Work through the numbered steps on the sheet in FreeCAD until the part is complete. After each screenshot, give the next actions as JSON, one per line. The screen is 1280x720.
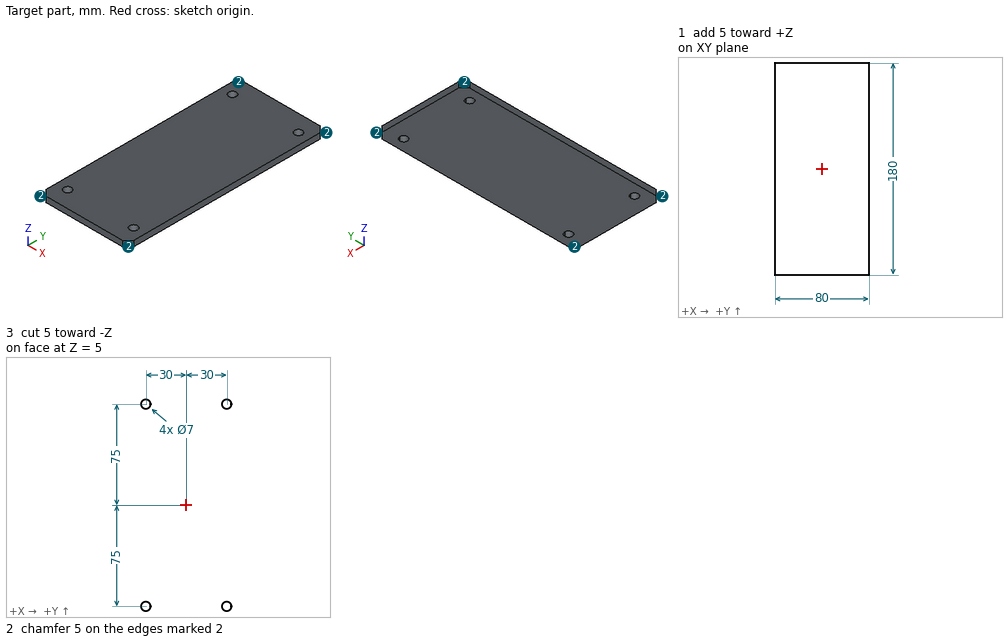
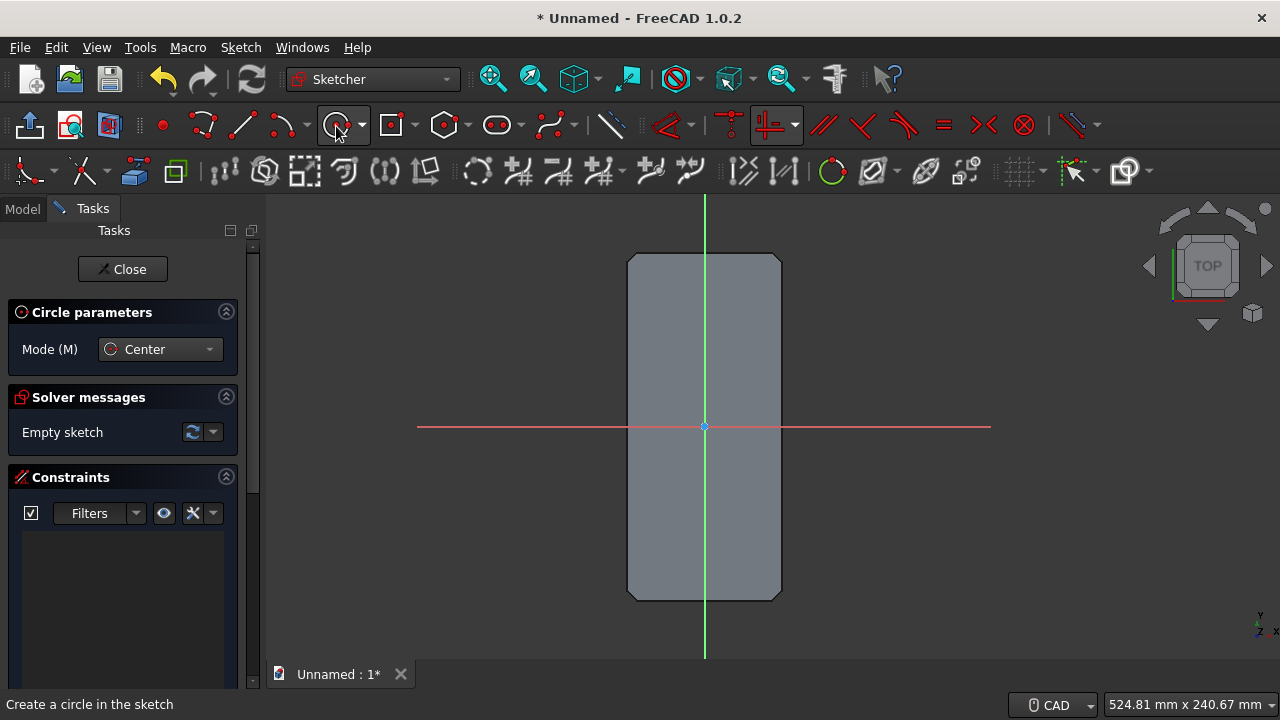
{"action": "scroll", "coordinate": [647, 282], "scroll_direction": "up", "scroll_amount": 7}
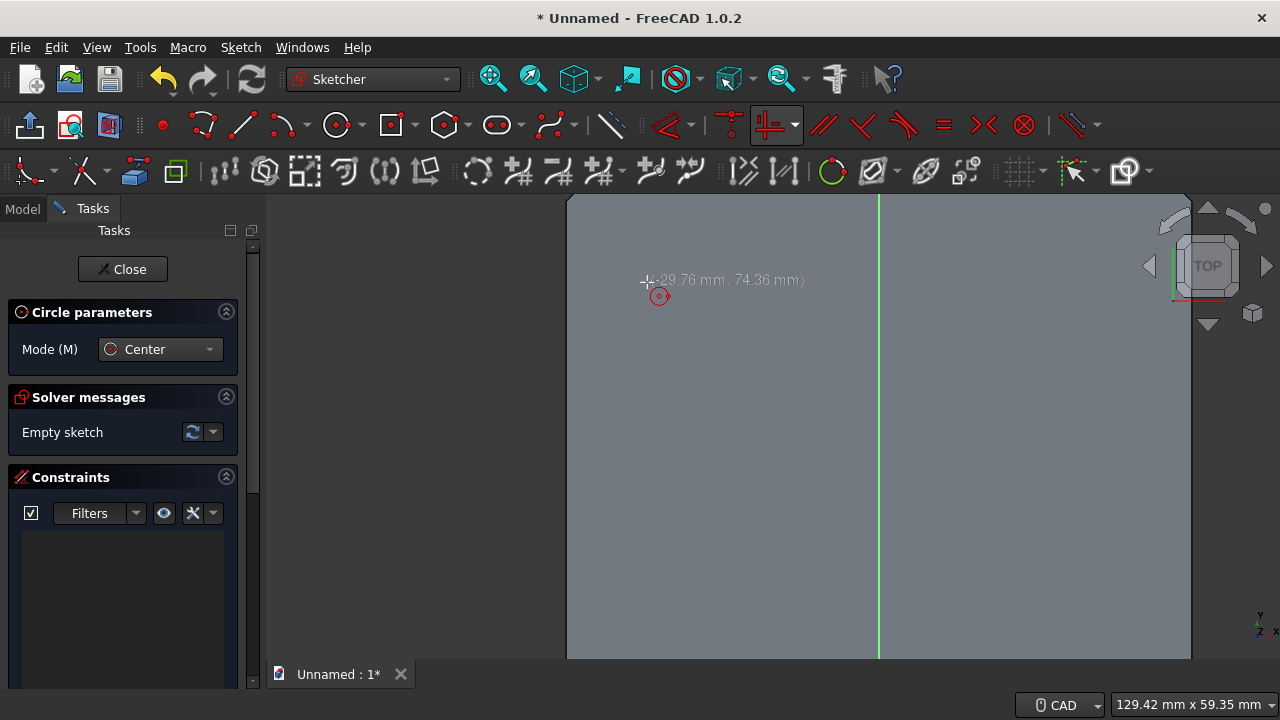
{"action": "scroll", "coordinate": [647, 282], "scroll_direction": "down", "scroll_amount": 7}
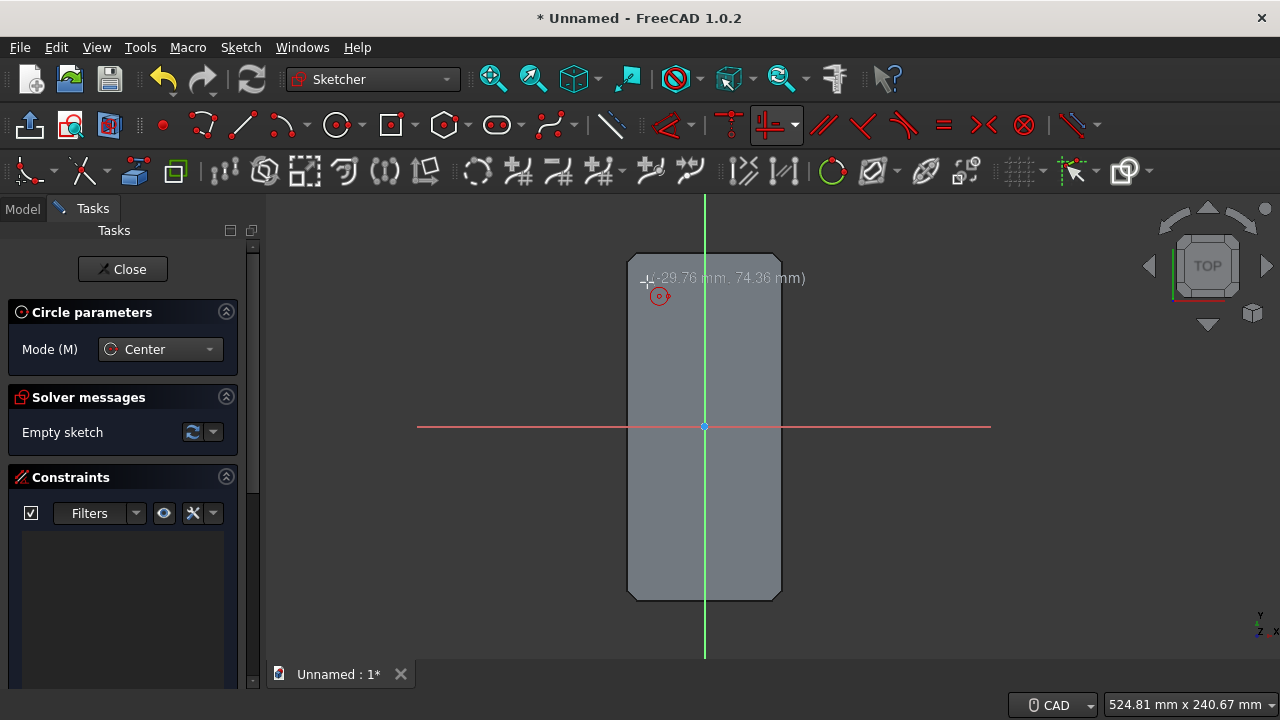
{"action": "left_click", "coordinate": [647, 282]}
{"action": "mouse_move", "coordinate": [651, 277]}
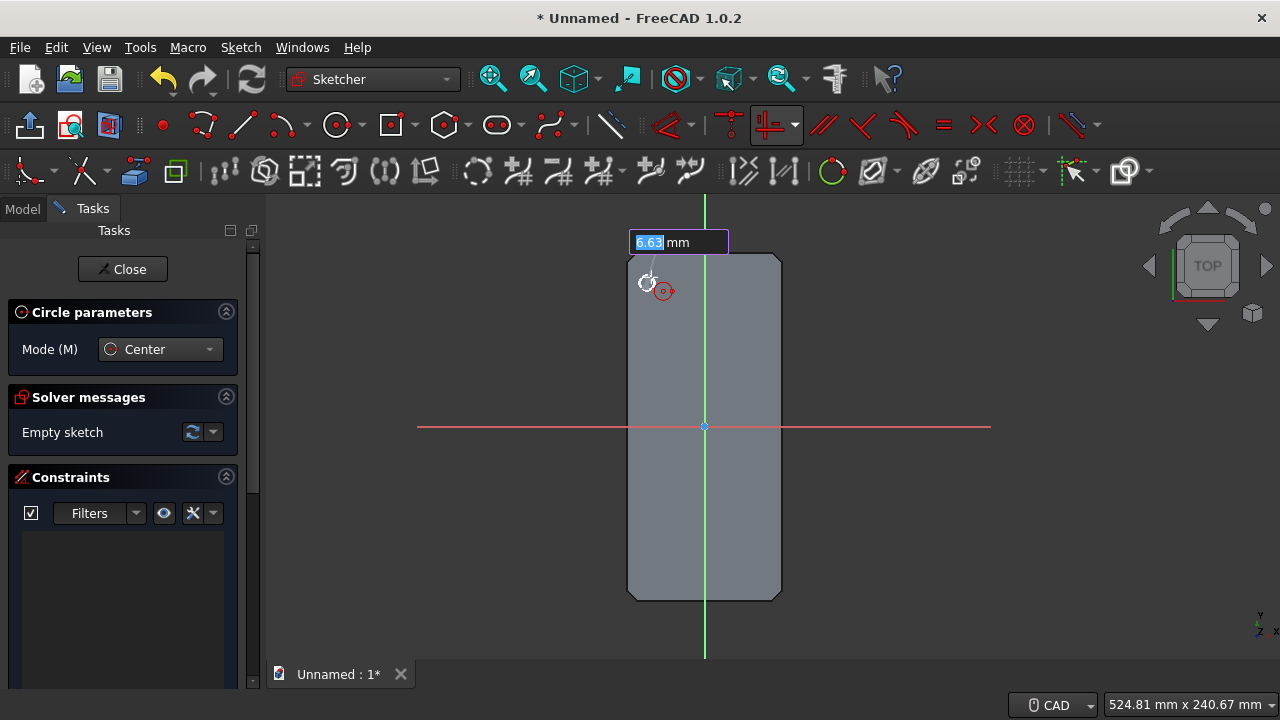
{"action": "type", "text": "7"}
{"action": "key", "text": "Return"}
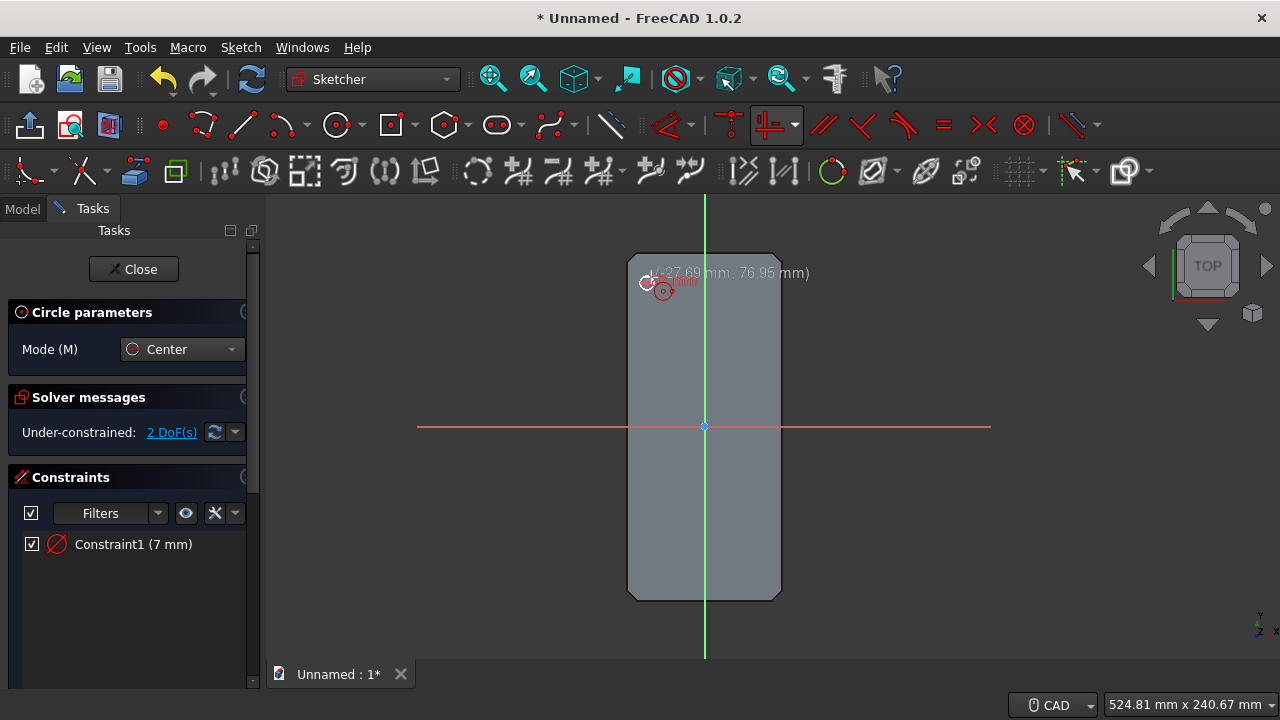
{"action": "scroll", "coordinate": [762, 282], "scroll_direction": "up", "scroll_amount": 7}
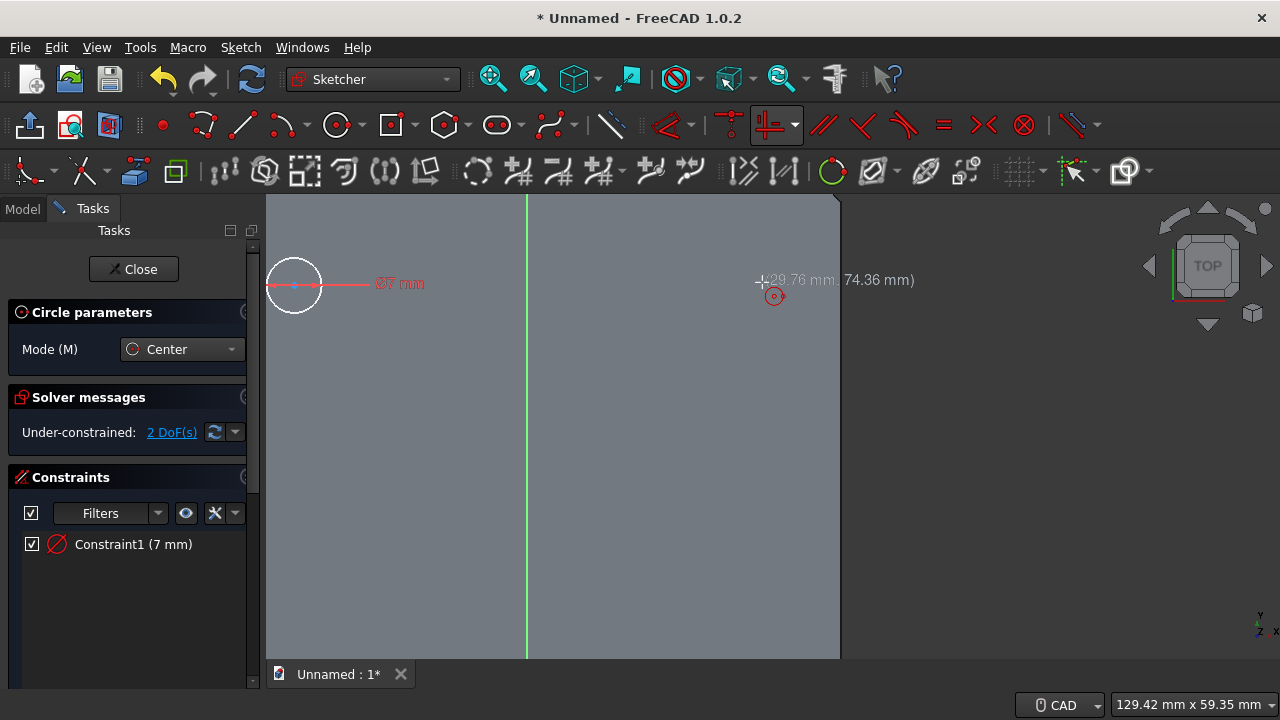
{"action": "scroll", "coordinate": [762, 282], "scroll_direction": "down", "scroll_amount": 7}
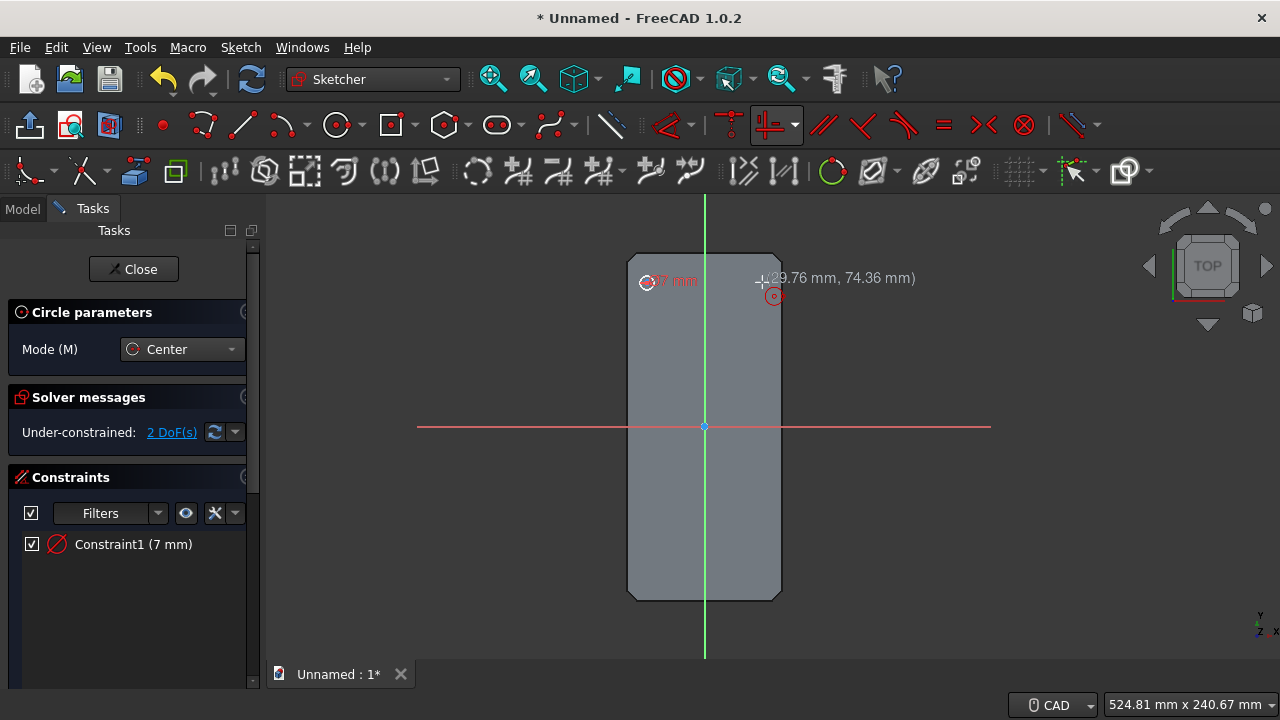
{"action": "left_click", "coordinate": [762, 282]}
{"action": "mouse_move", "coordinate": [767, 277]}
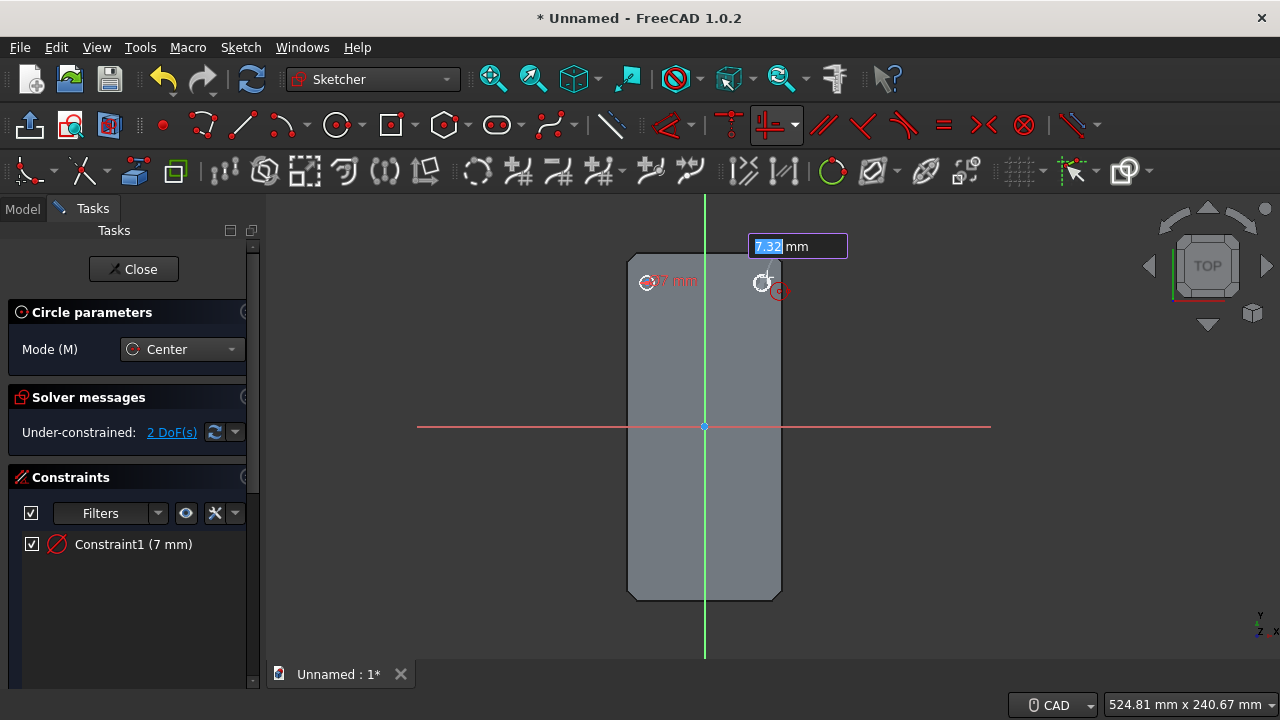
{"action": "type", "text": "7"}
{"action": "key", "text": "Return"}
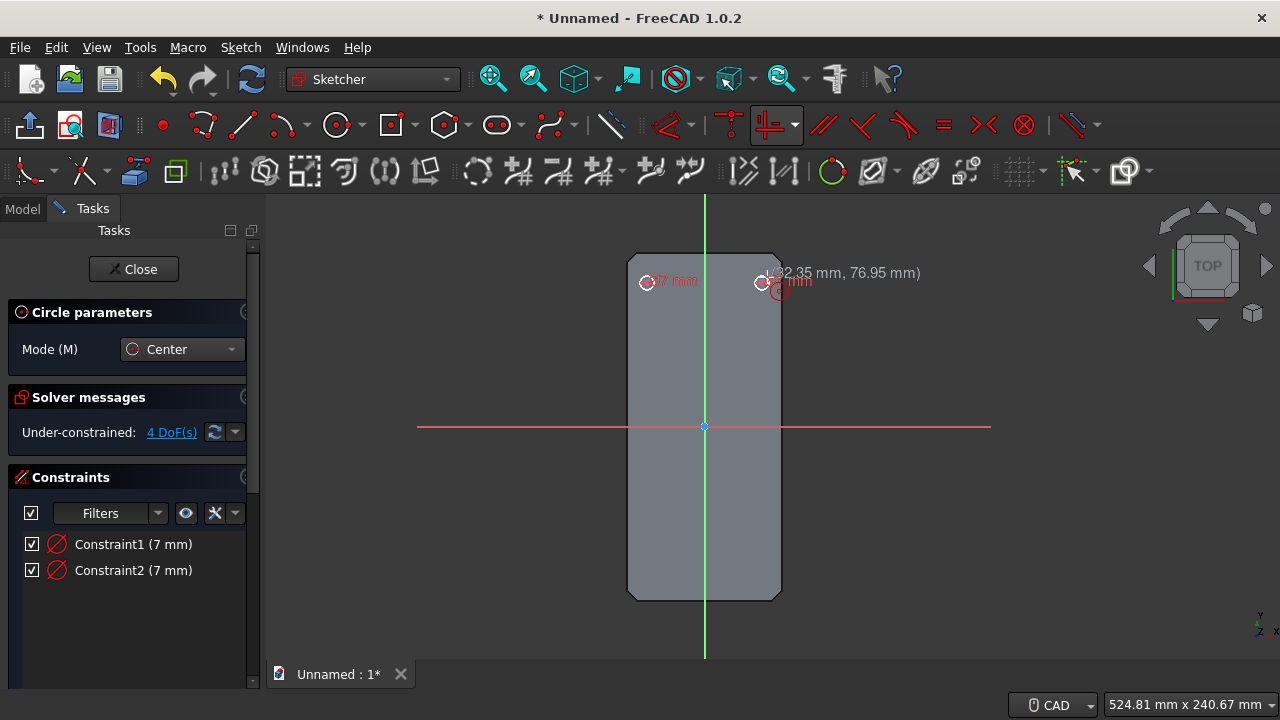
{"action": "scroll", "coordinate": [647, 572], "scroll_direction": "up", "scroll_amount": 7}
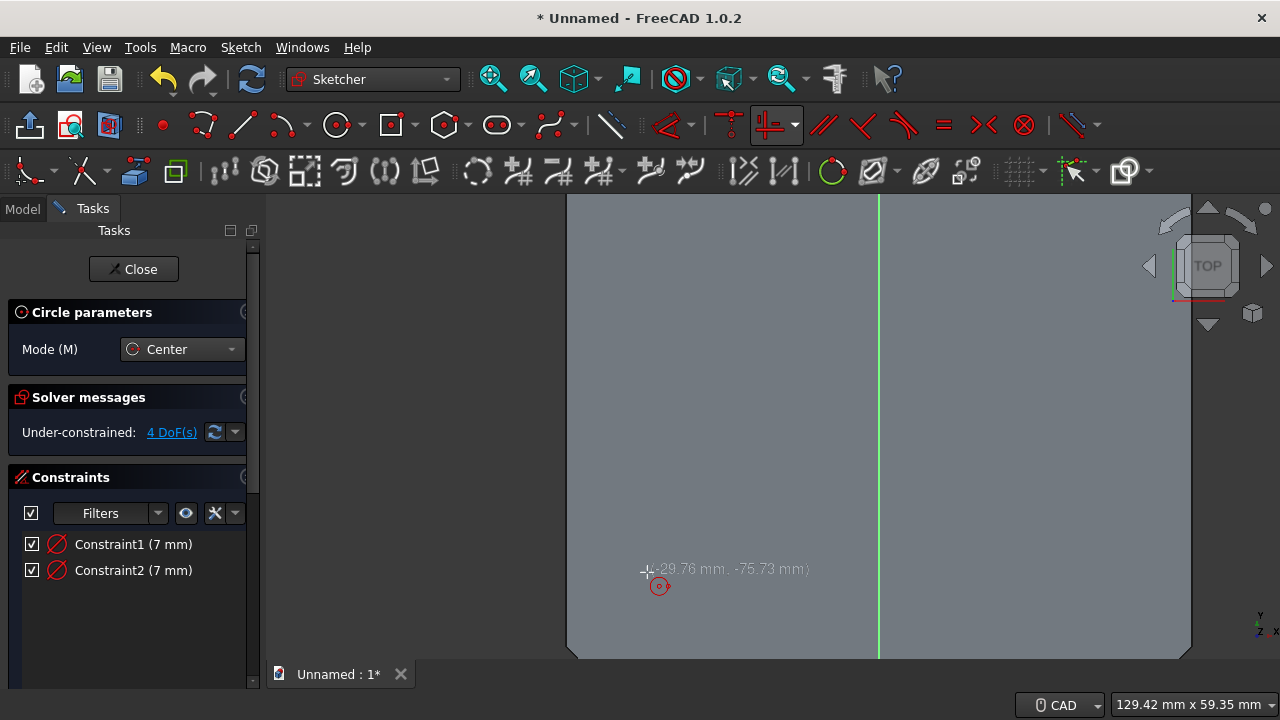
{"action": "scroll", "coordinate": [647, 573], "scroll_direction": "down", "scroll_amount": 7}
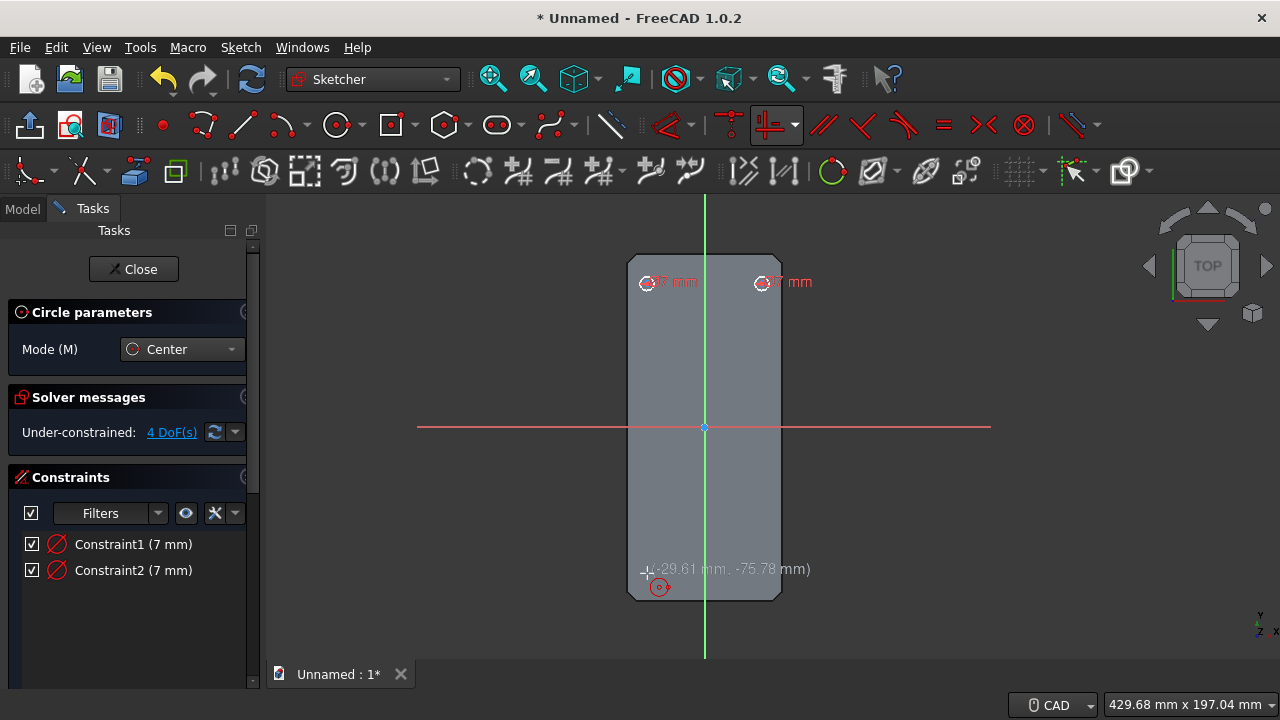
{"action": "left_click", "coordinate": [647, 572]}
{"action": "mouse_move", "coordinate": [651, 568]}